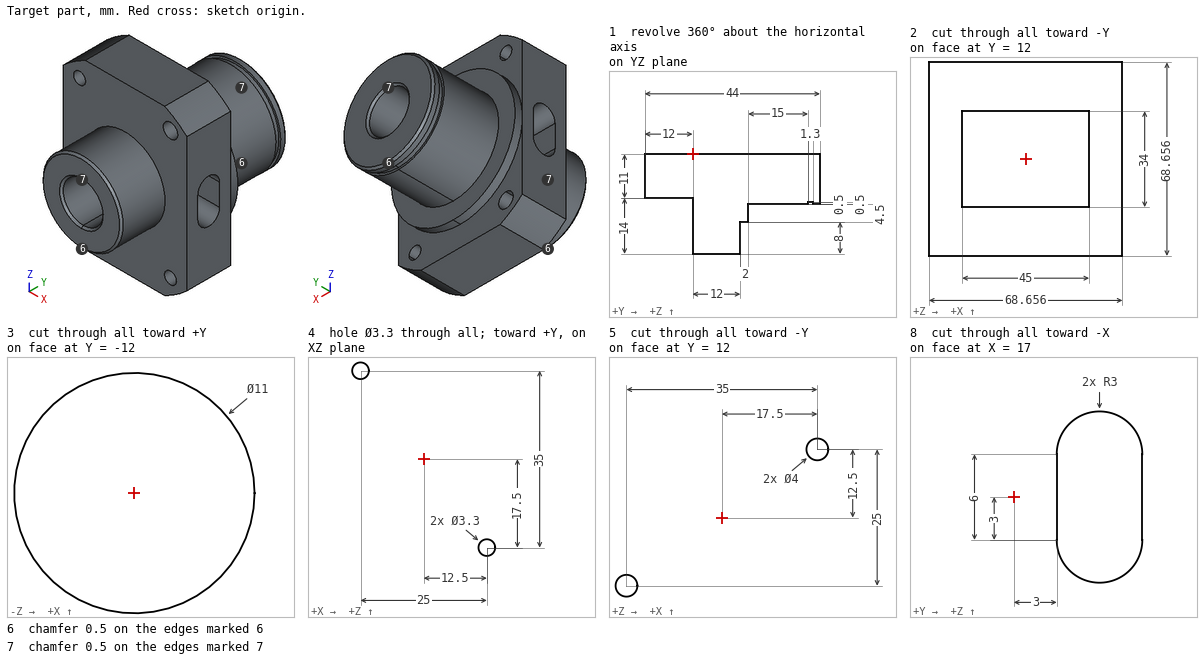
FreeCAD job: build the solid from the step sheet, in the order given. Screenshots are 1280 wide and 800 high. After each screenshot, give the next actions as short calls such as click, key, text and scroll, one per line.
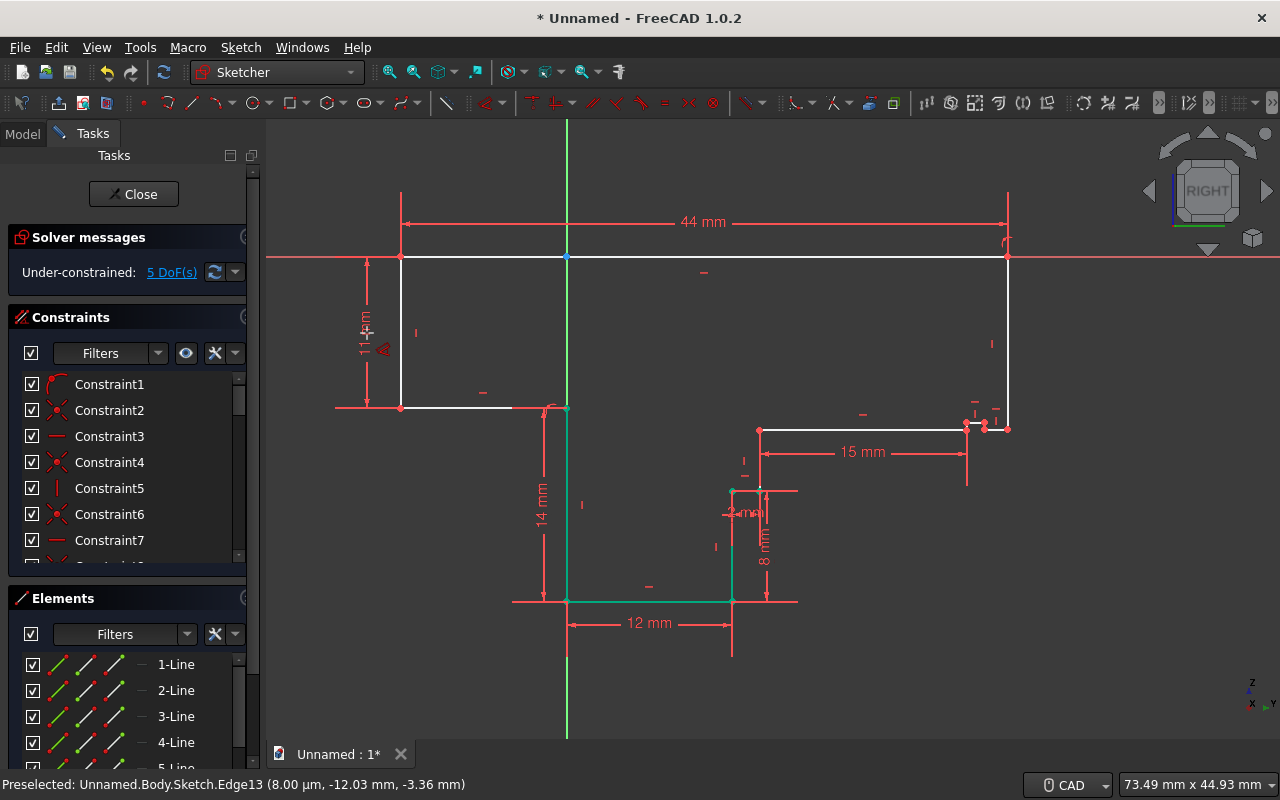
click(450, 408)
click(484, 374)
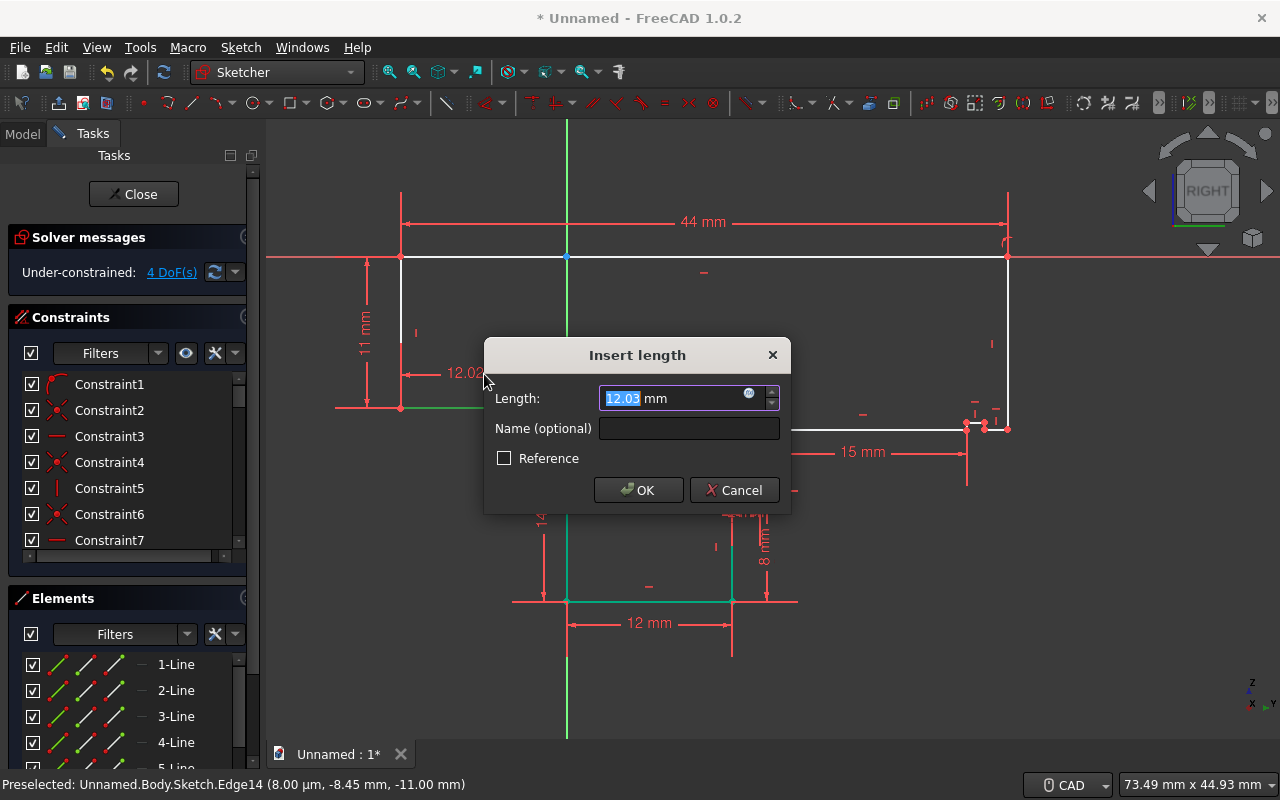
text(12)
key(Return)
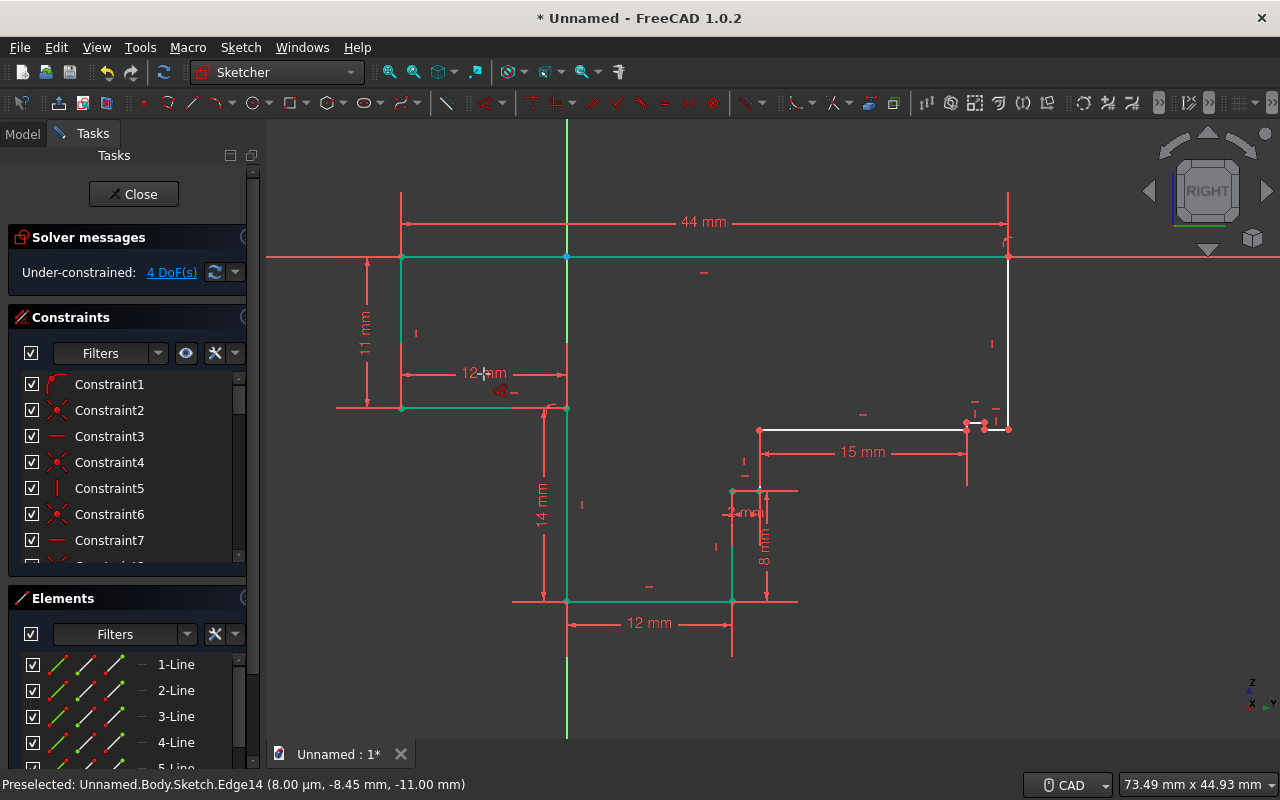
click(760, 473)
click(794, 475)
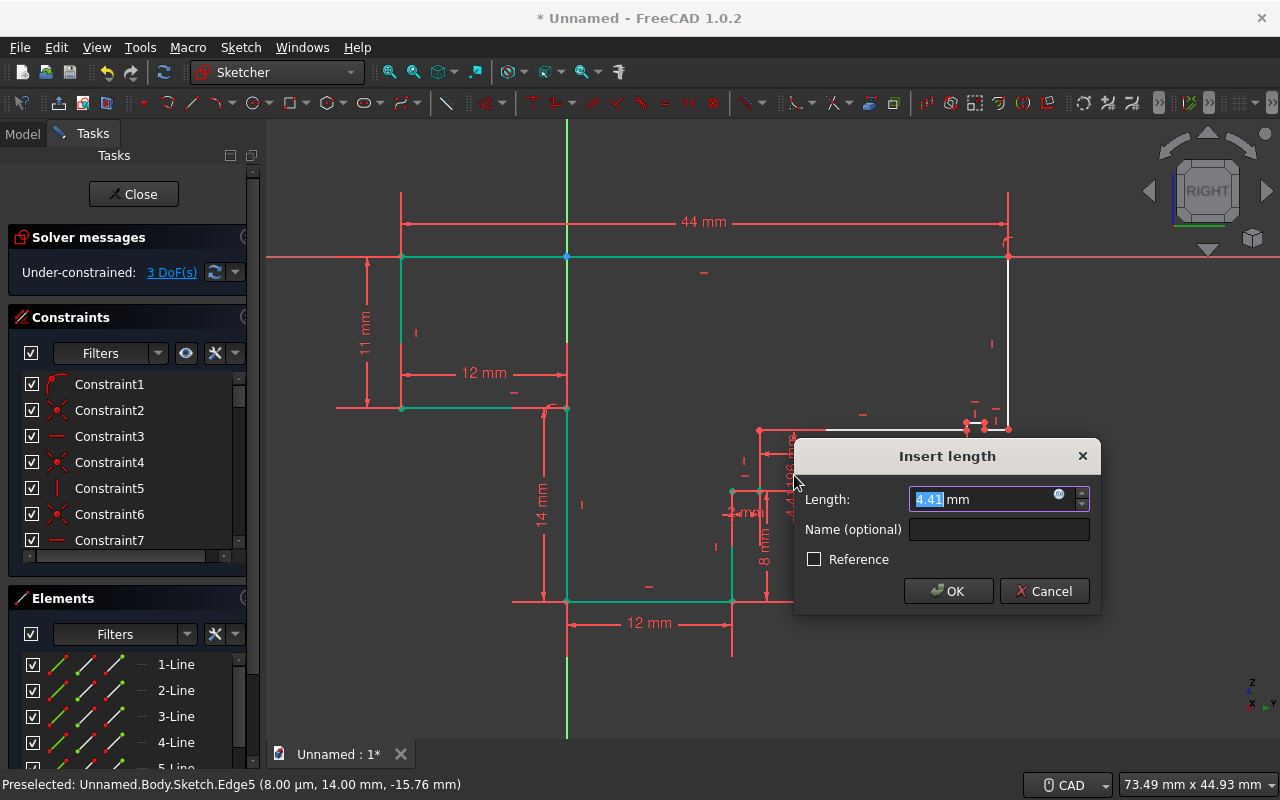
text(4.5)
key(Return)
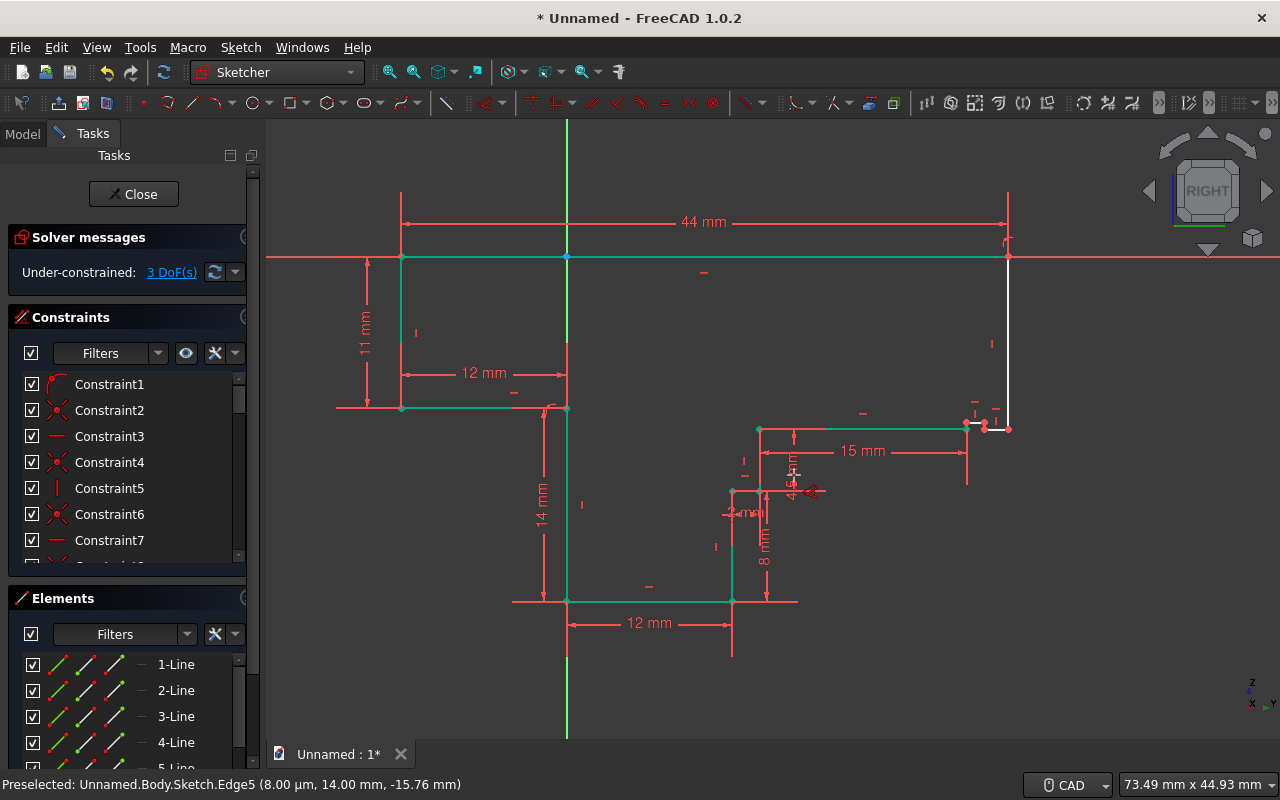
scroll(967, 426, up, 9)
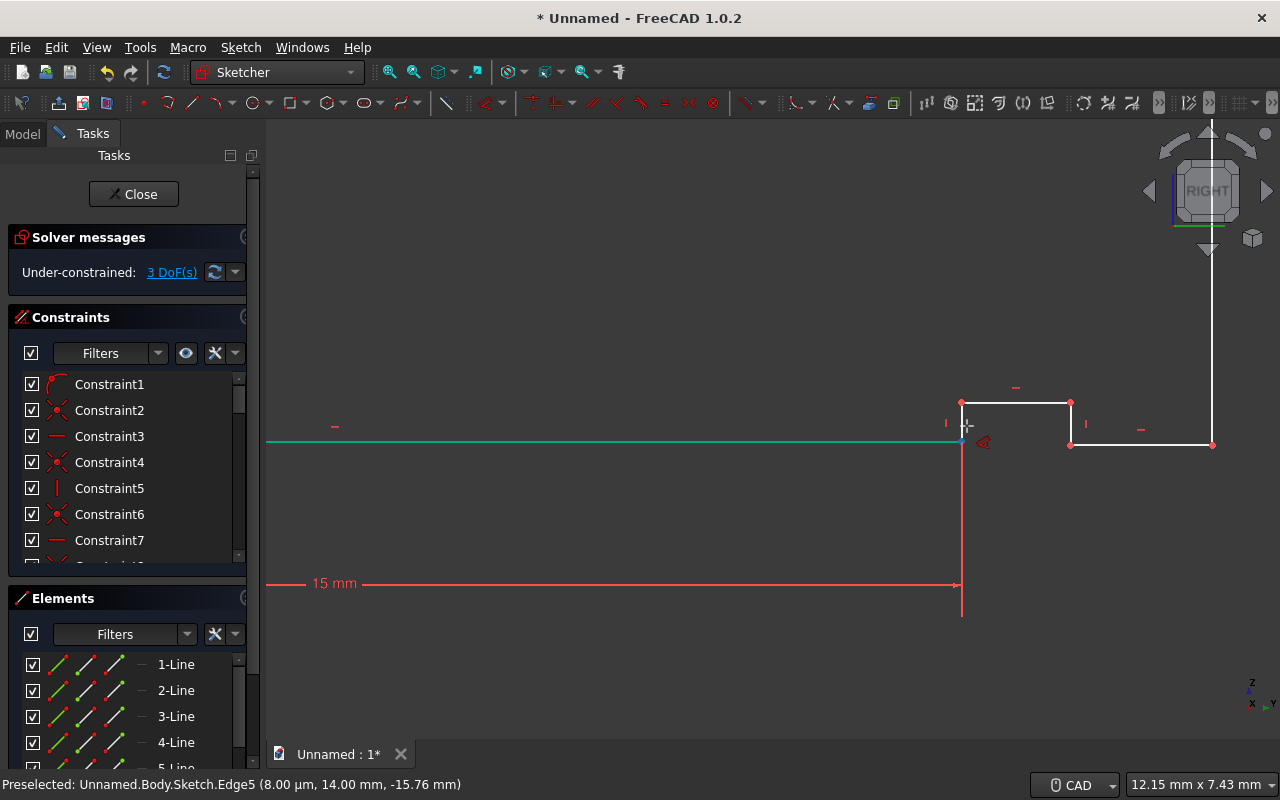
click(962, 422)
click(996, 422)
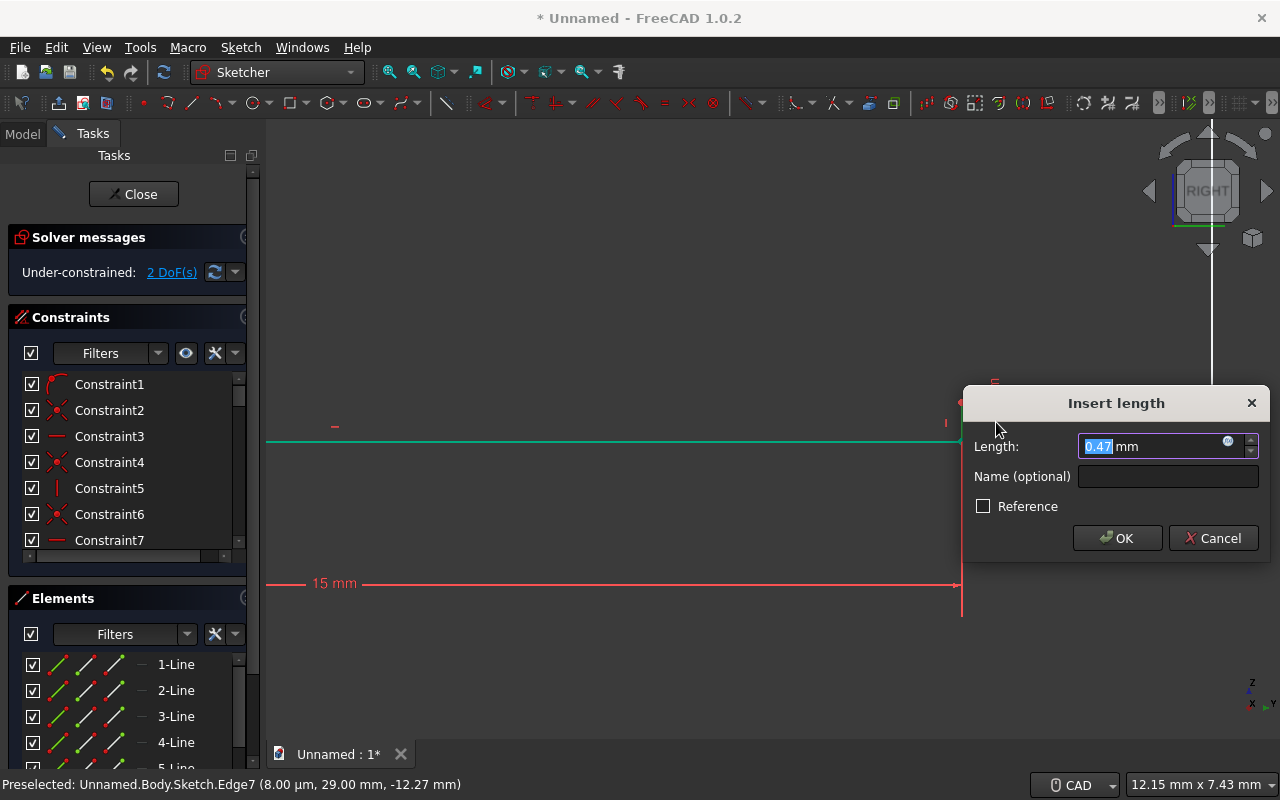
text(0.5)
key(Return)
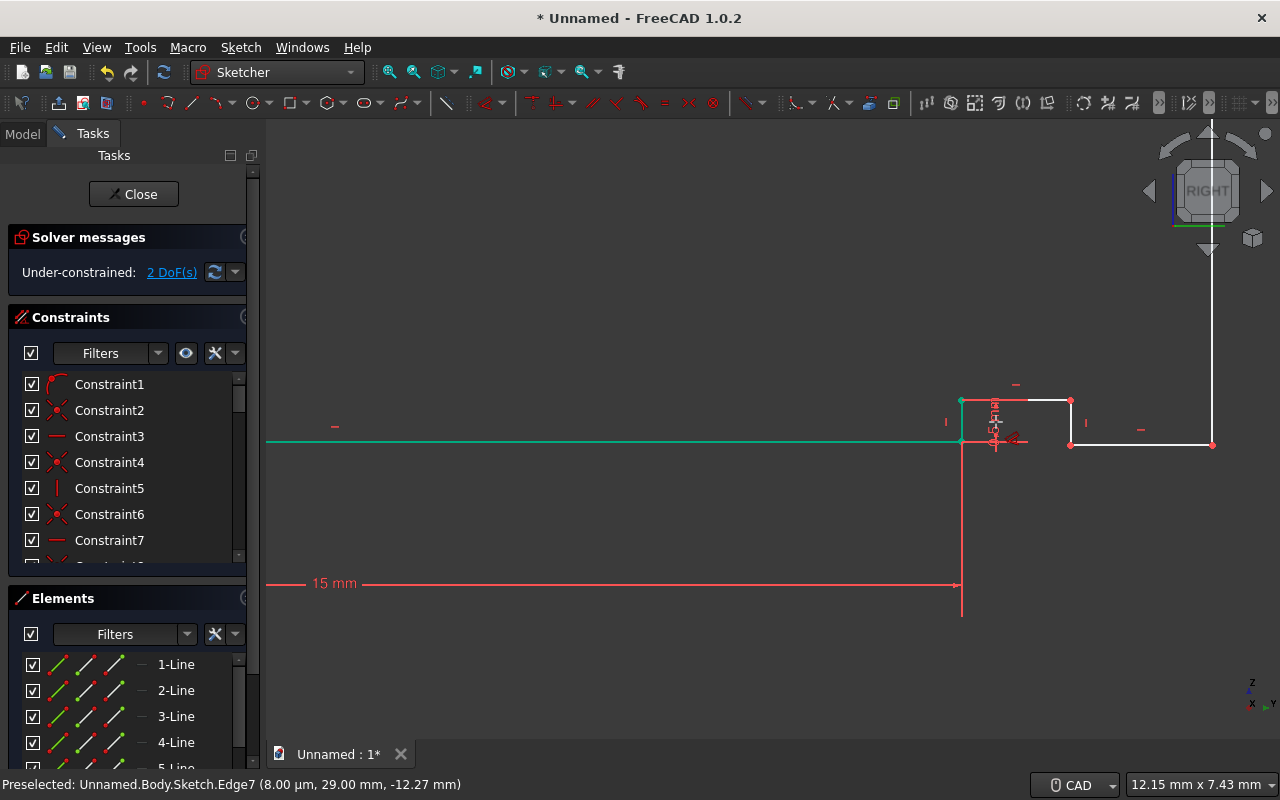
click(995, 400)
click(1016, 366)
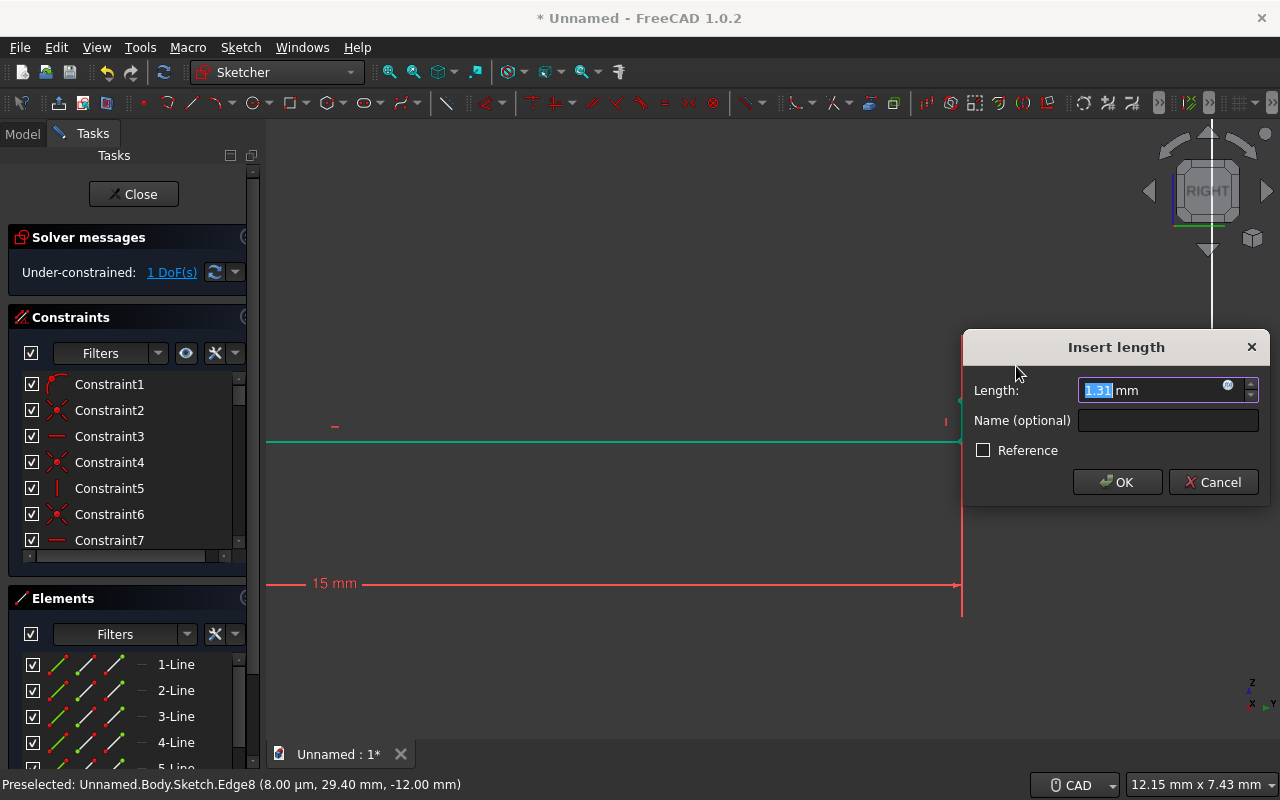
text(1.3)
key(Return)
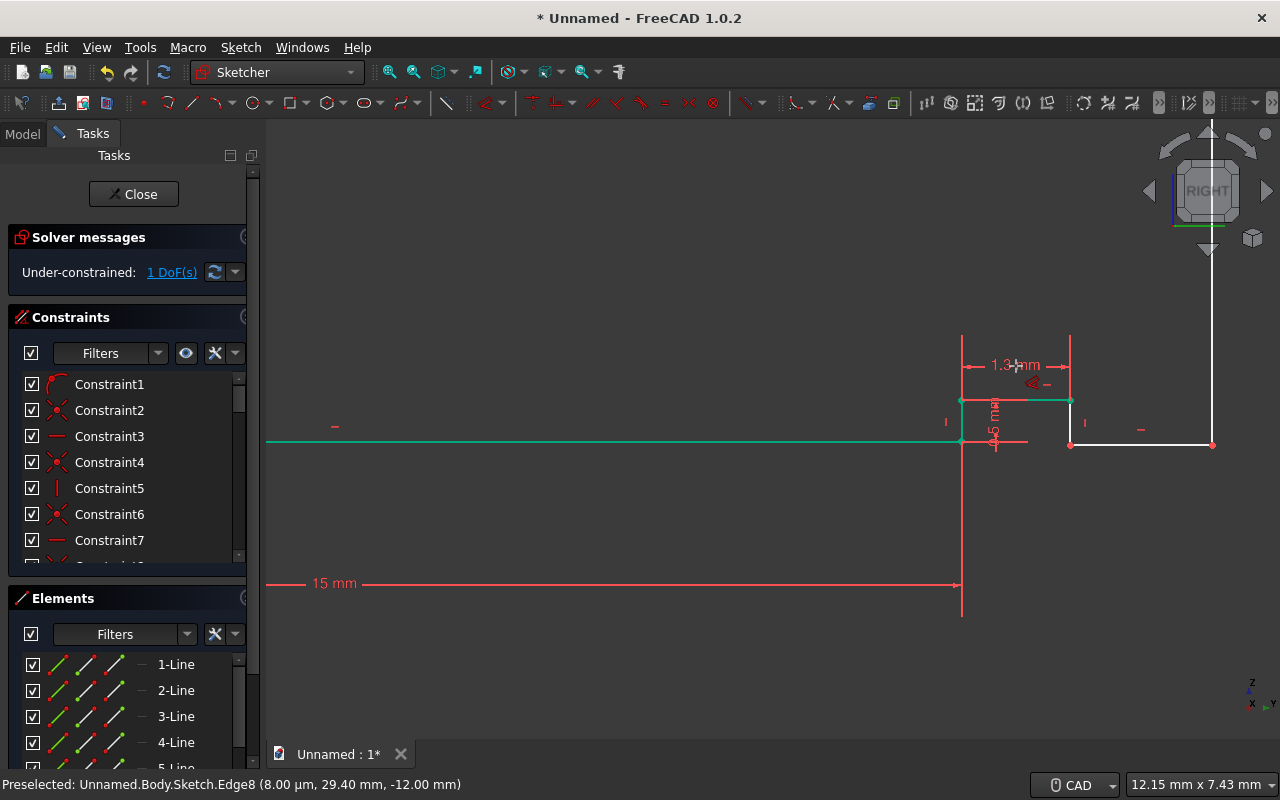
click(1070, 414)
click(1104, 423)